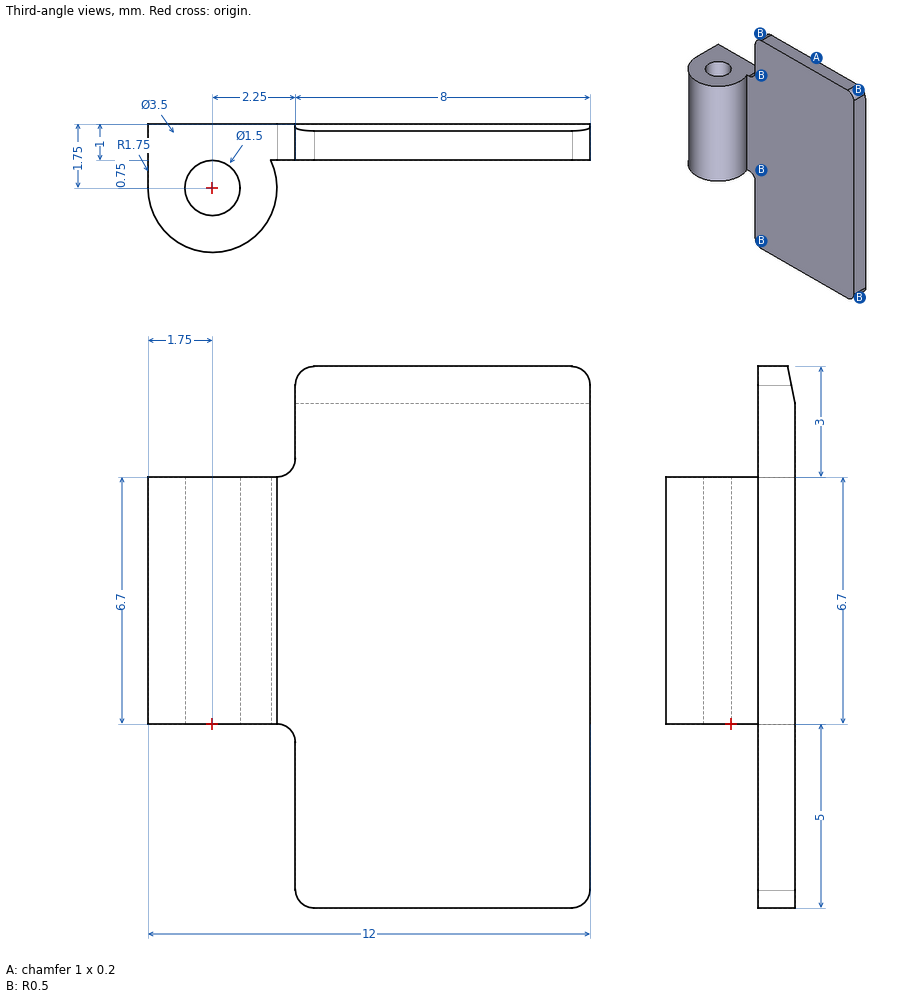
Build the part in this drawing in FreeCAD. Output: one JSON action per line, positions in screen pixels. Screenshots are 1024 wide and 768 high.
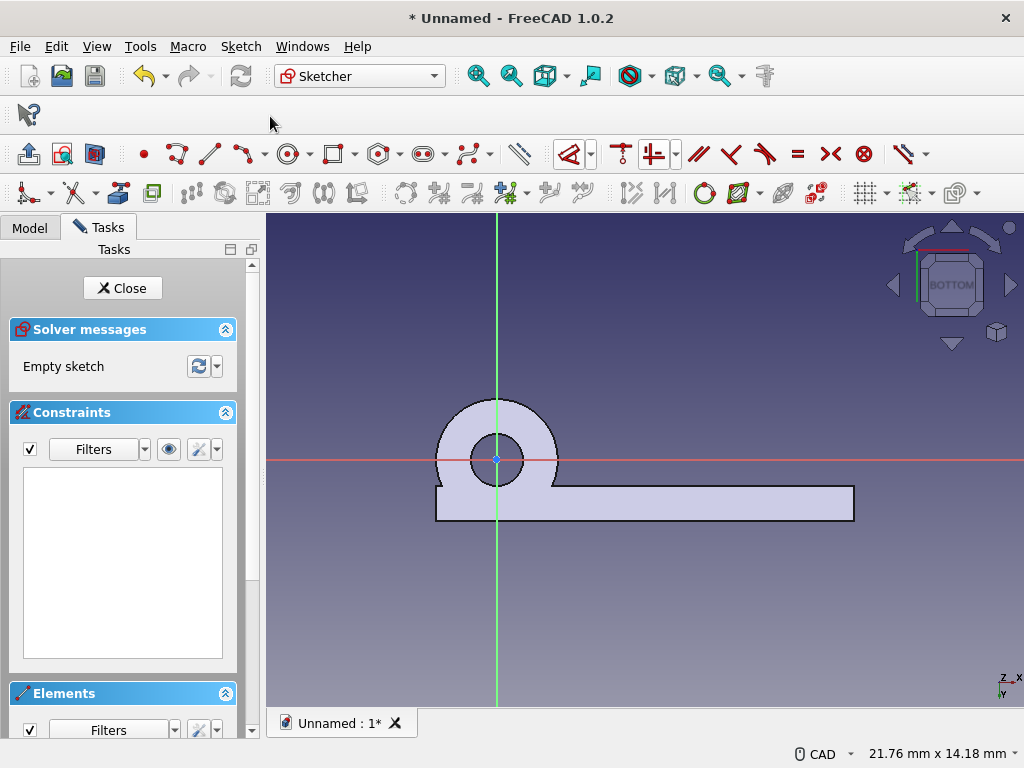
{"action": "scroll", "coordinate": [445, 476], "scroll_direction": "up", "scroll_amount": 9}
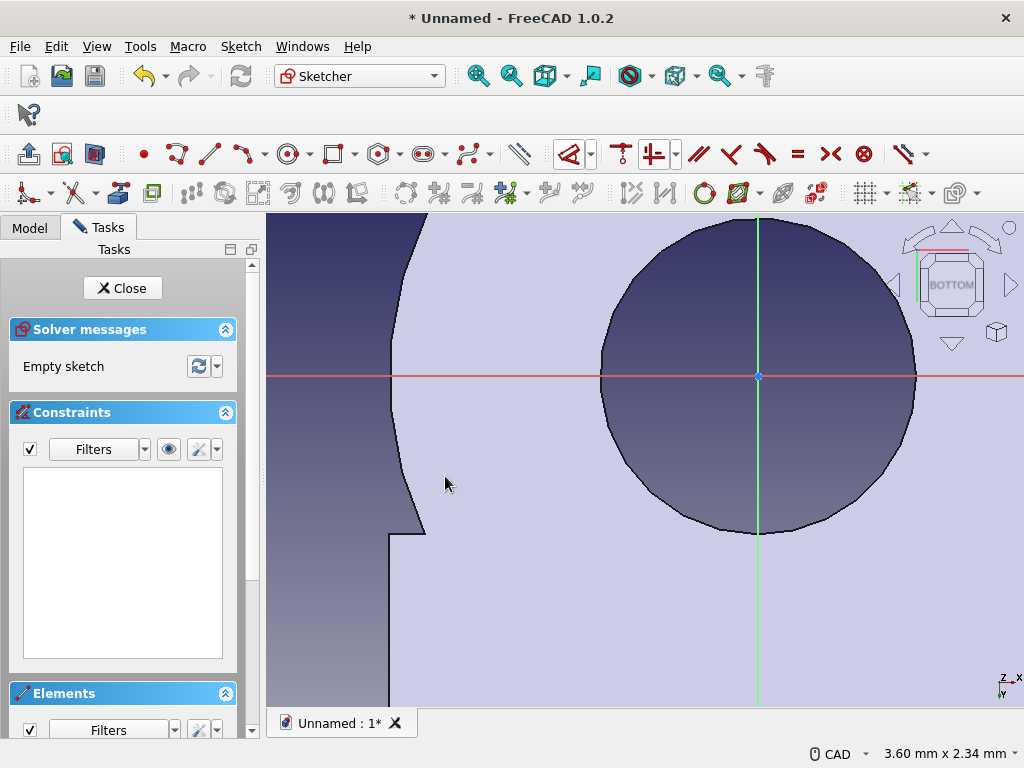
{"action": "key", "text": "g m"}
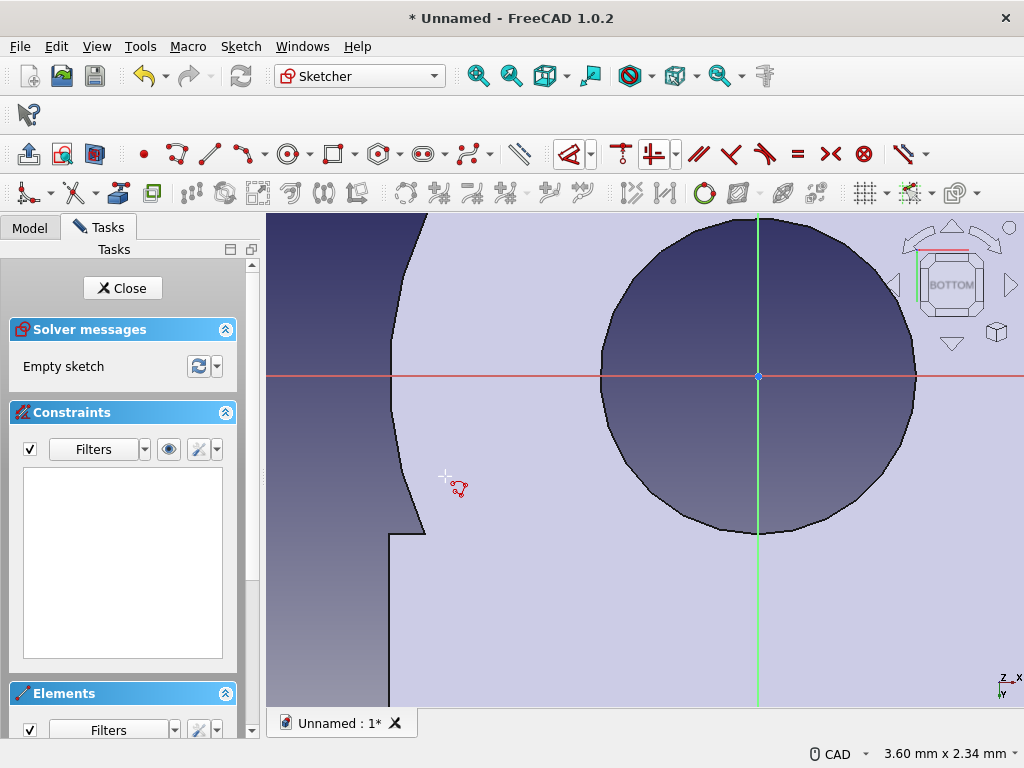
{"action": "left_click", "coordinate": [425, 534]}
{"action": "left_click", "coordinate": [389, 534]}
{"action": "left_click", "coordinate": [389, 376]}
{"action": "right_click", "coordinate": [389, 376]}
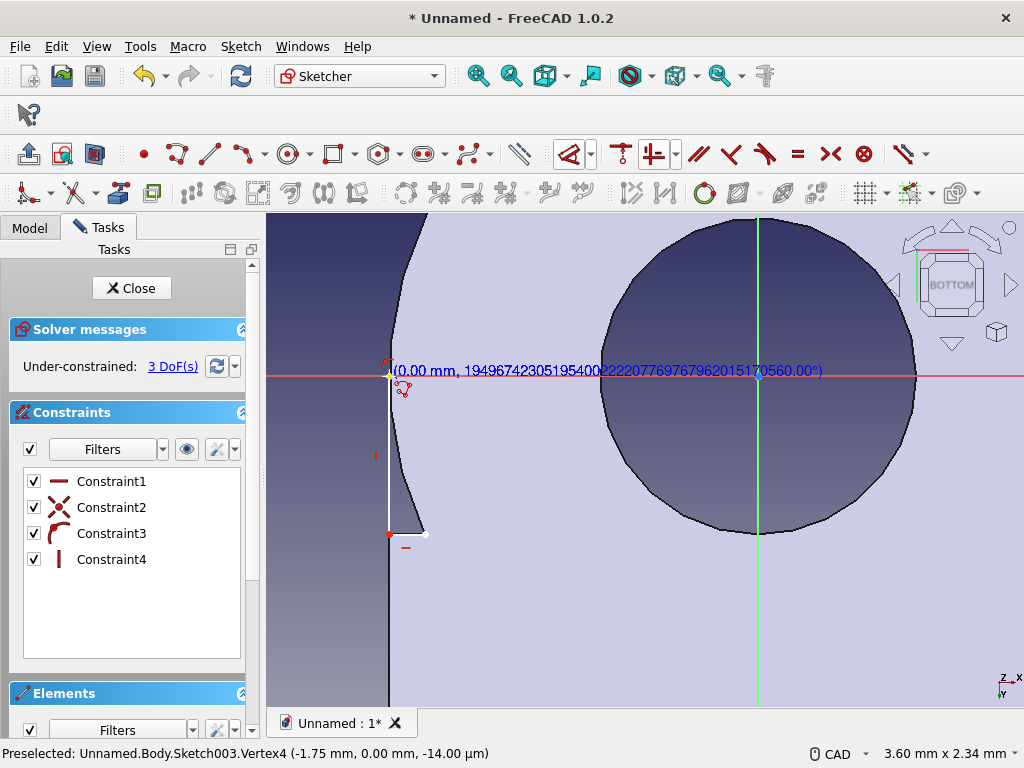
{"action": "left_click", "coordinate": [242, 154]}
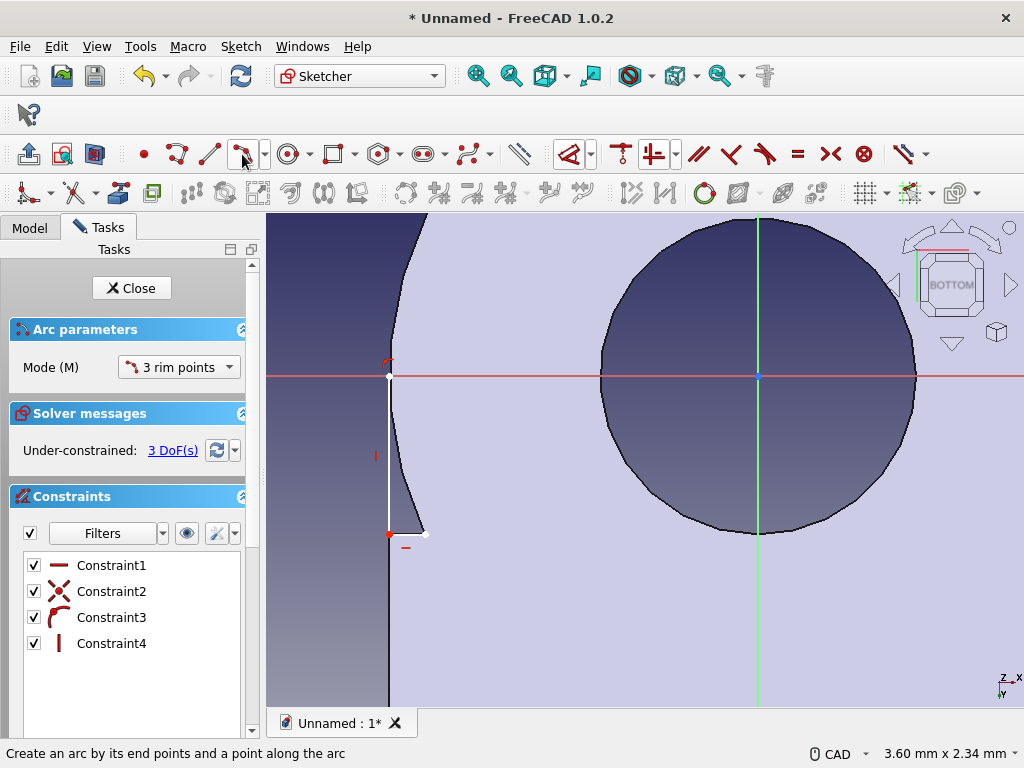
{"action": "left_click", "coordinate": [389, 376]}
{"action": "left_click", "coordinate": [425, 535]}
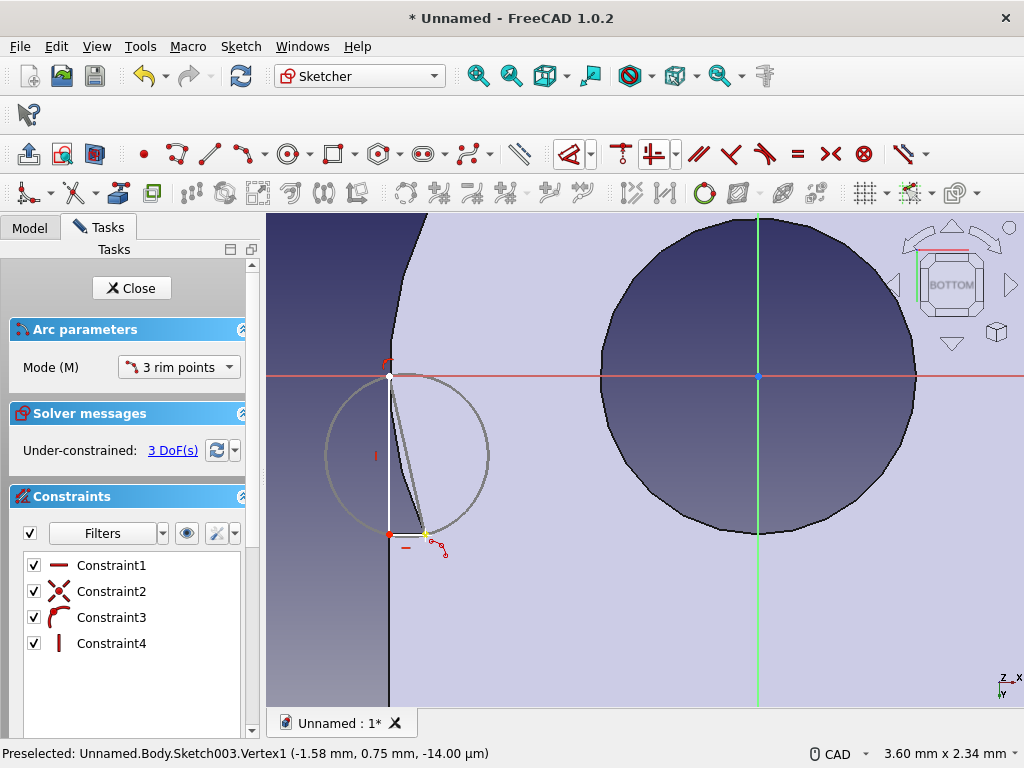
{"action": "scroll", "coordinate": [398, 457], "scroll_direction": "up", "scroll_amount": 3}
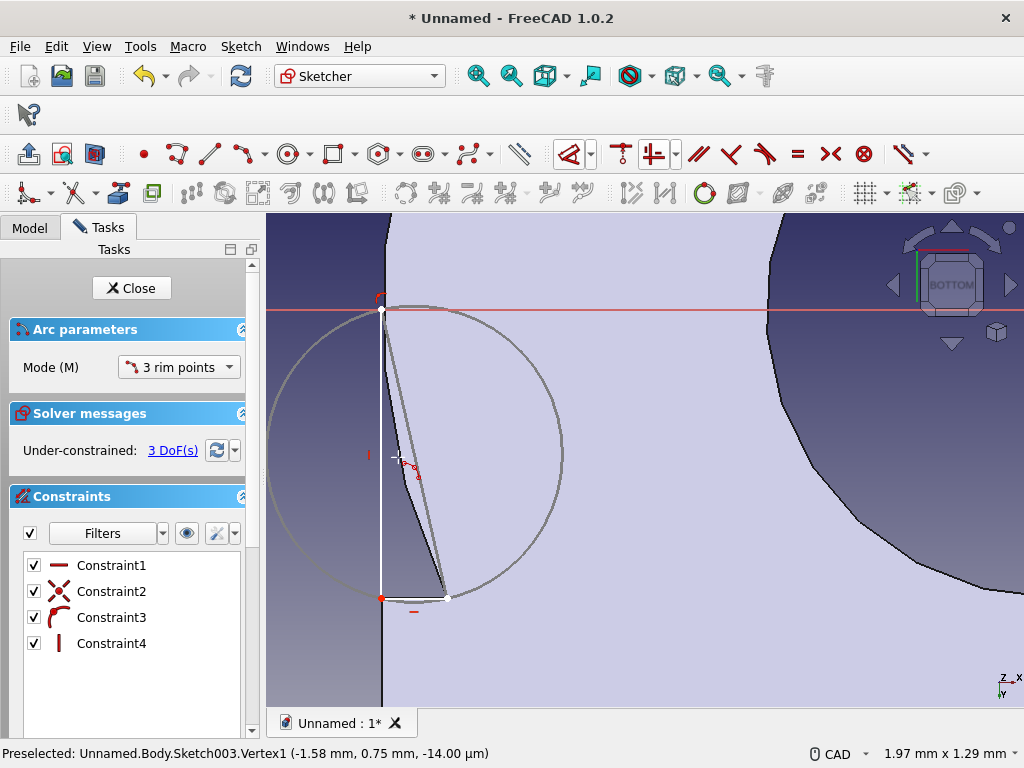
{"action": "left_click", "coordinate": [399, 457]}
{"action": "key", "text": "Escape"}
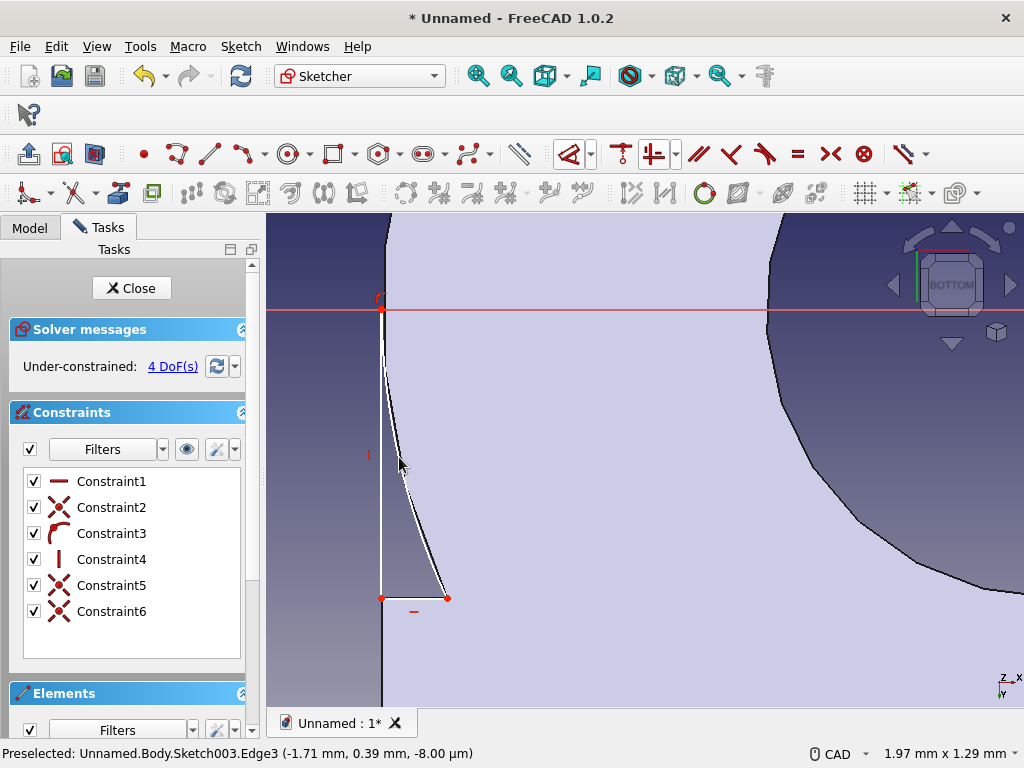
{"action": "left_click", "coordinate": [381, 512]}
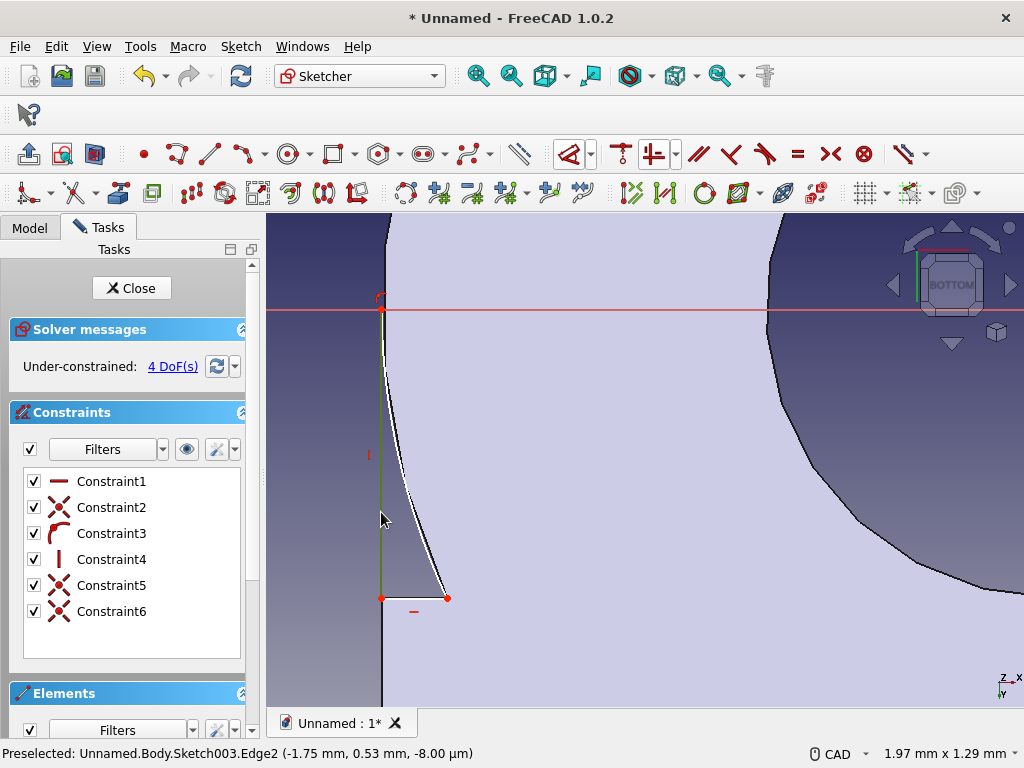
{"action": "left_click", "coordinate": [415, 515]}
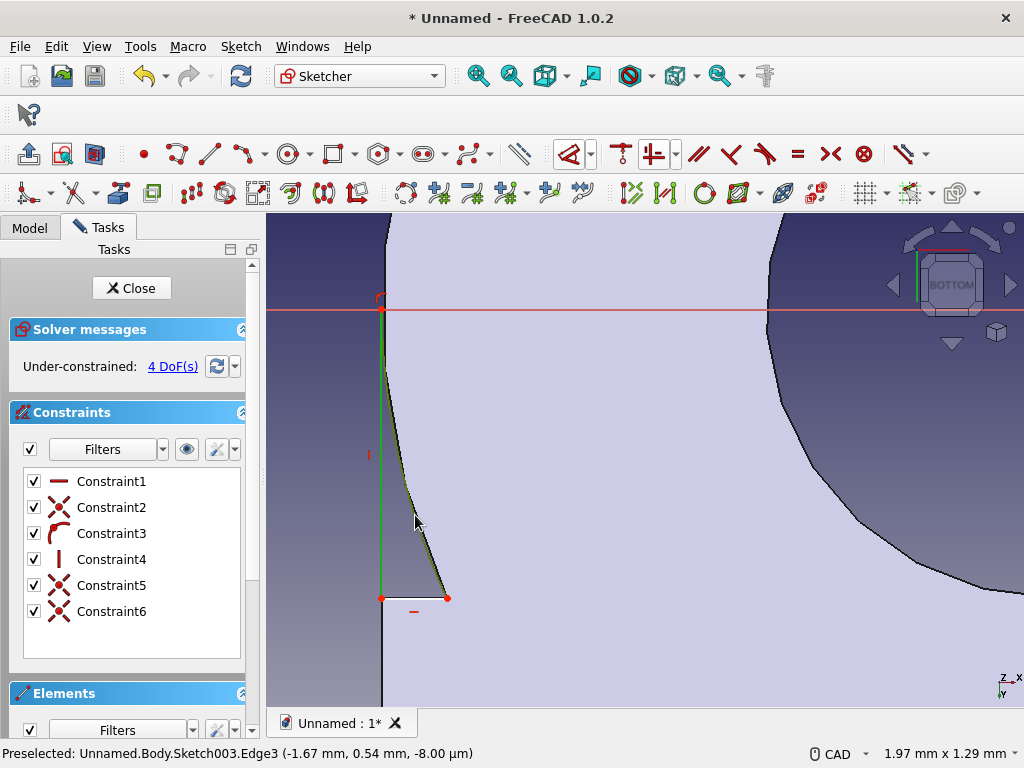
{"action": "left_click", "coordinate": [765, 154]}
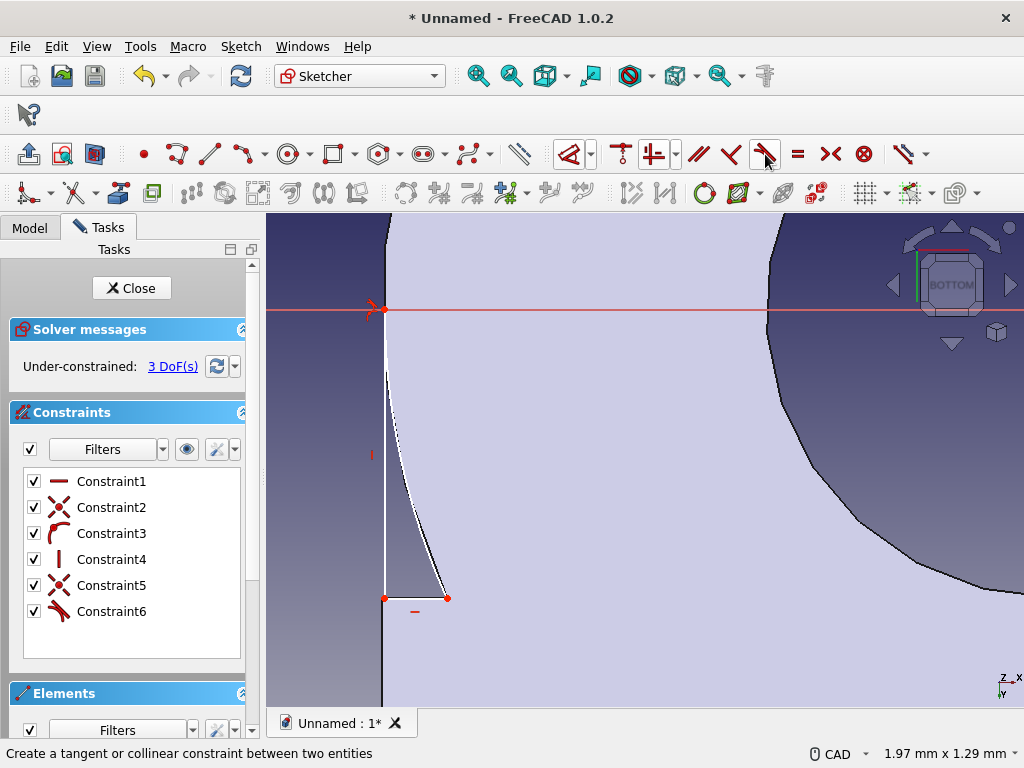
{"action": "scroll", "coordinate": [404, 468], "scroll_direction": "down", "scroll_amount": 3}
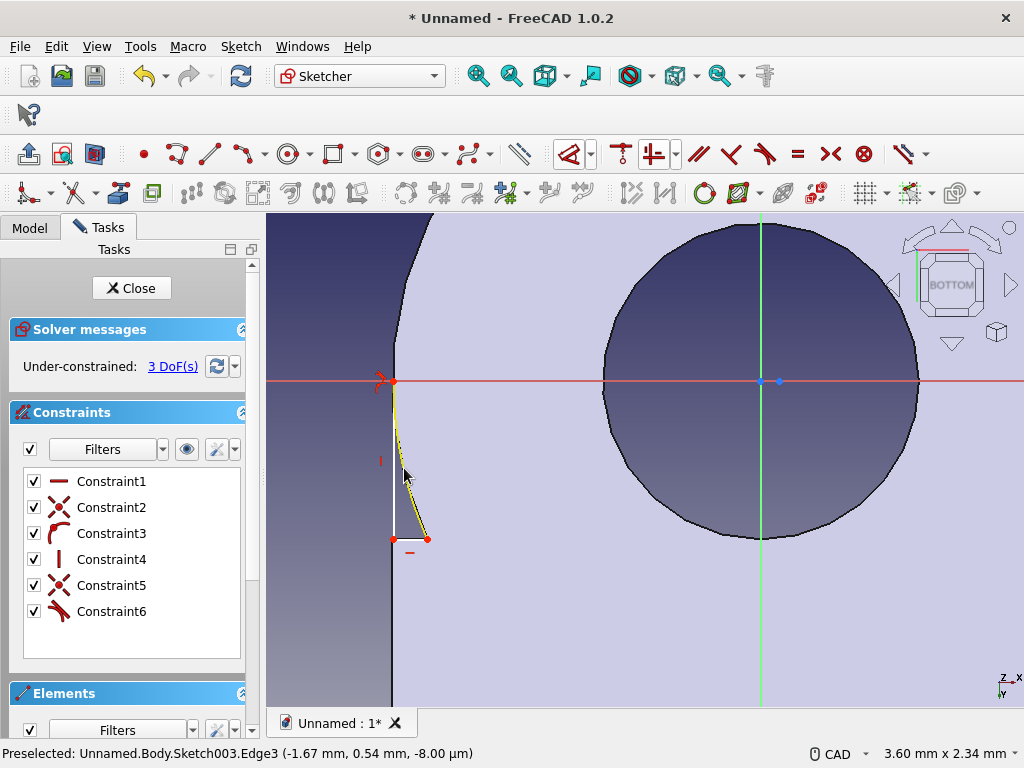
{"action": "left_click", "coordinate": [779, 381]}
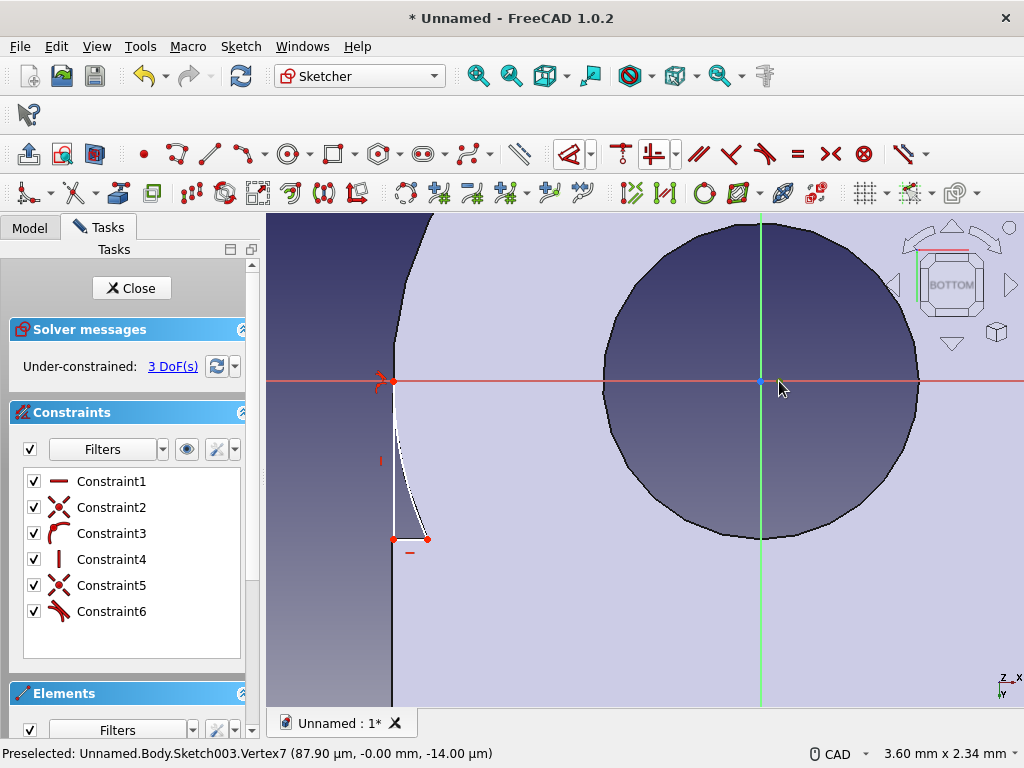
{"action": "left_click", "coordinate": [761, 648]}